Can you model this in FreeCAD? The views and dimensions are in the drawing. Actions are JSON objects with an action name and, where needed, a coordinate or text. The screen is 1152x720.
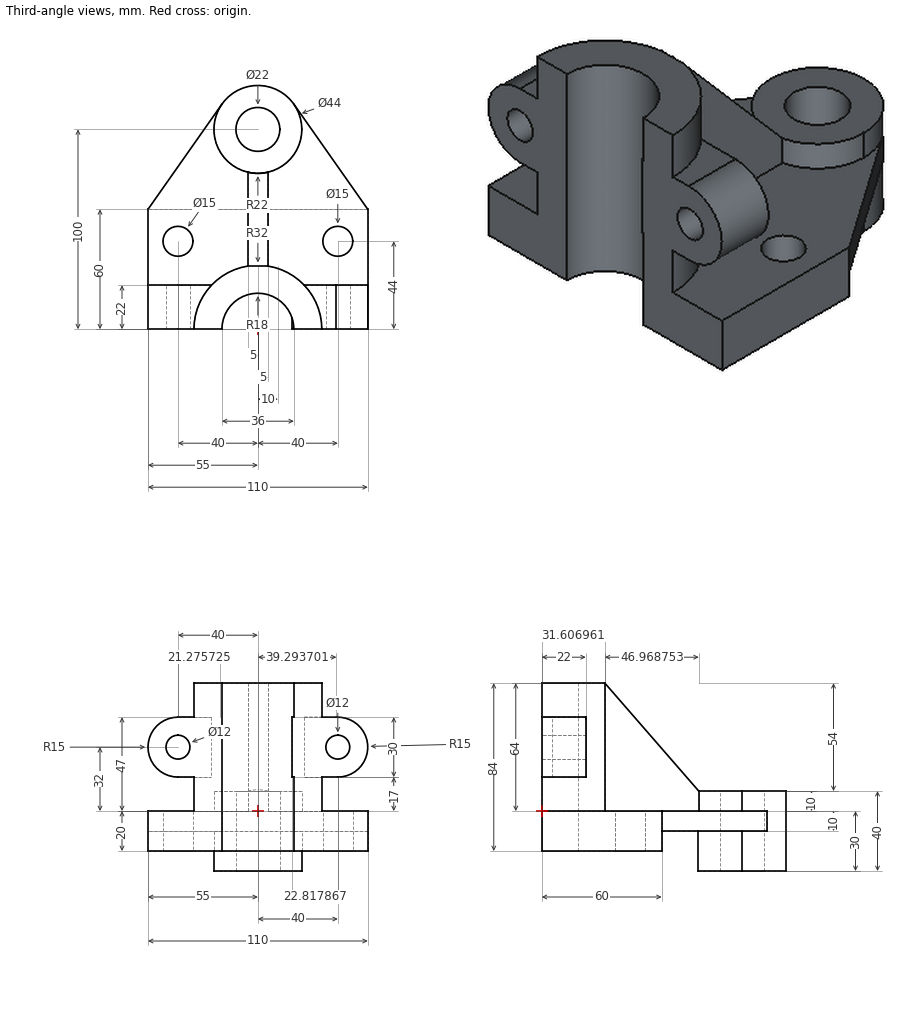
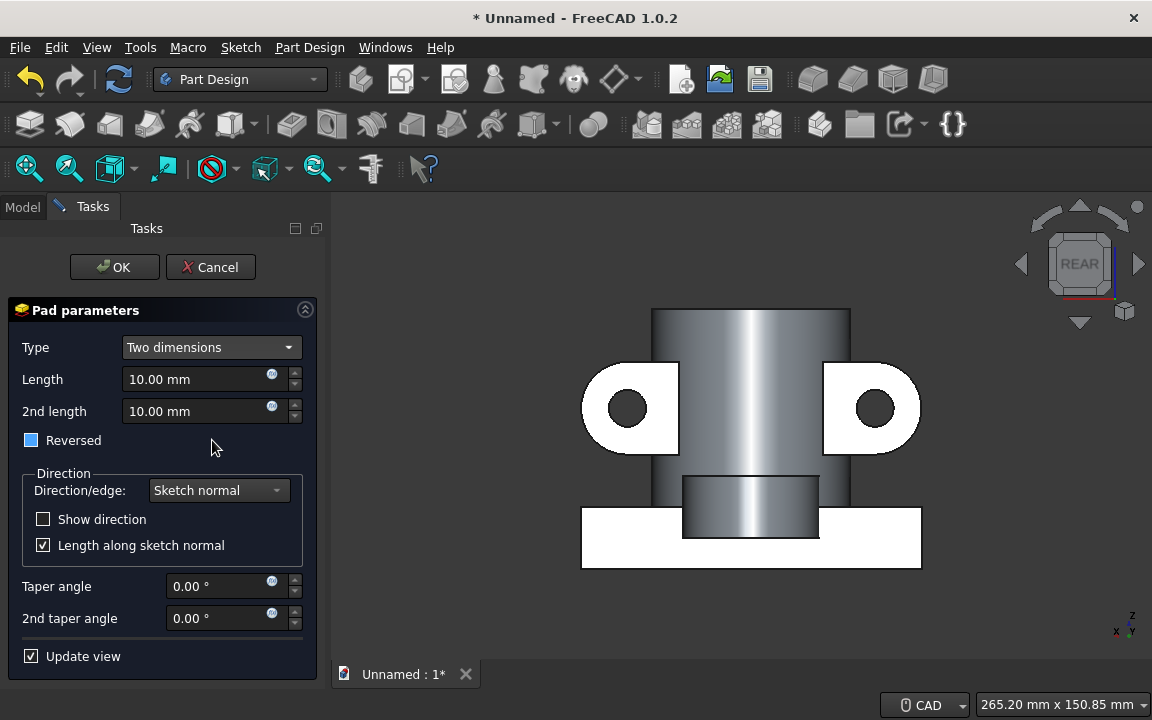
{"action": "triple_click", "coordinate": [204, 379]}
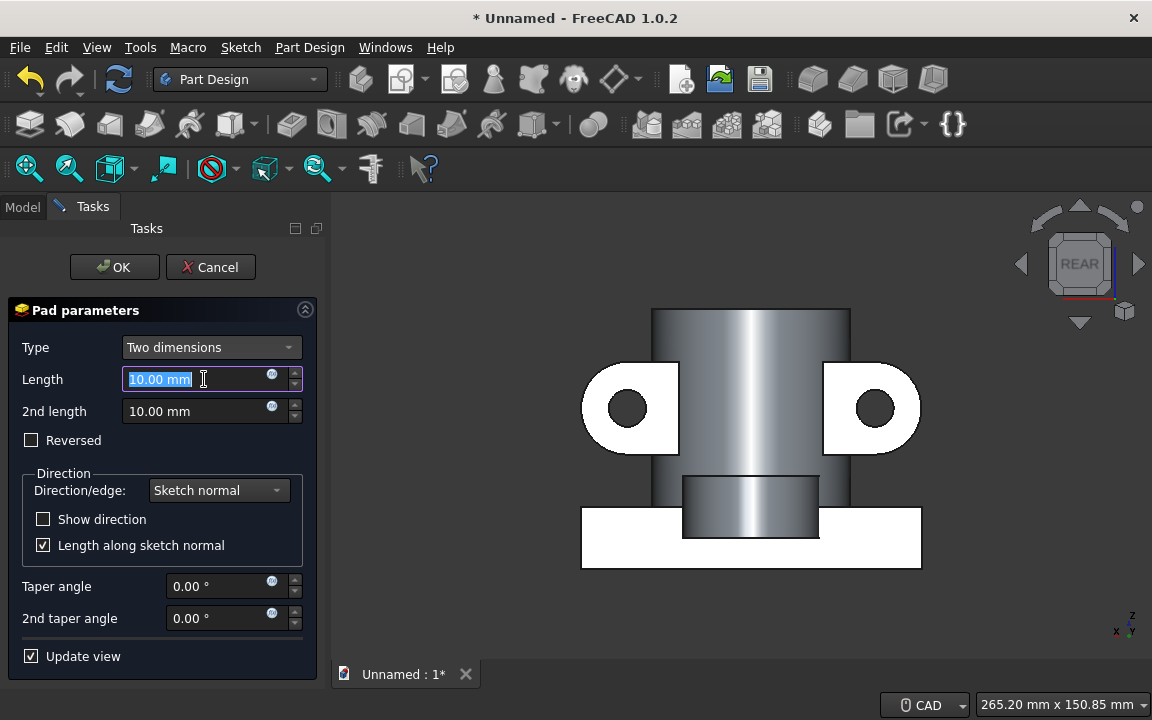
{"action": "type", "text": "10"}
{"action": "key", "text": "Tab"}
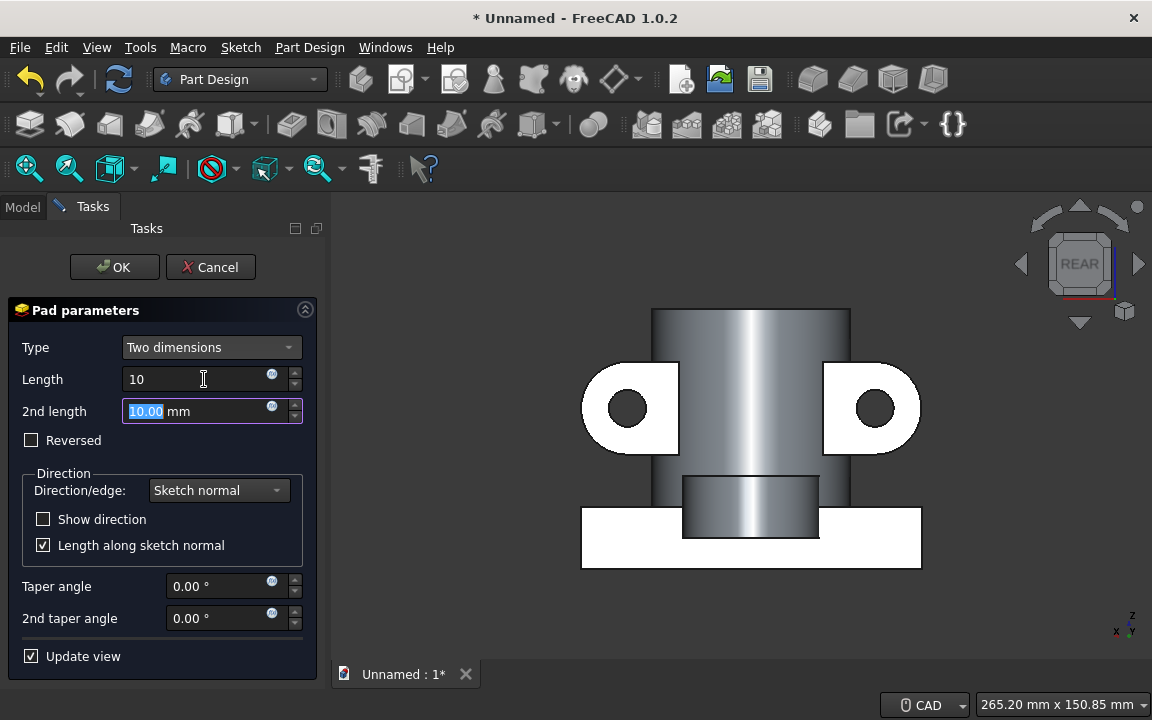
{"action": "type", "text": "30"}
{"action": "key", "text": "Tab"}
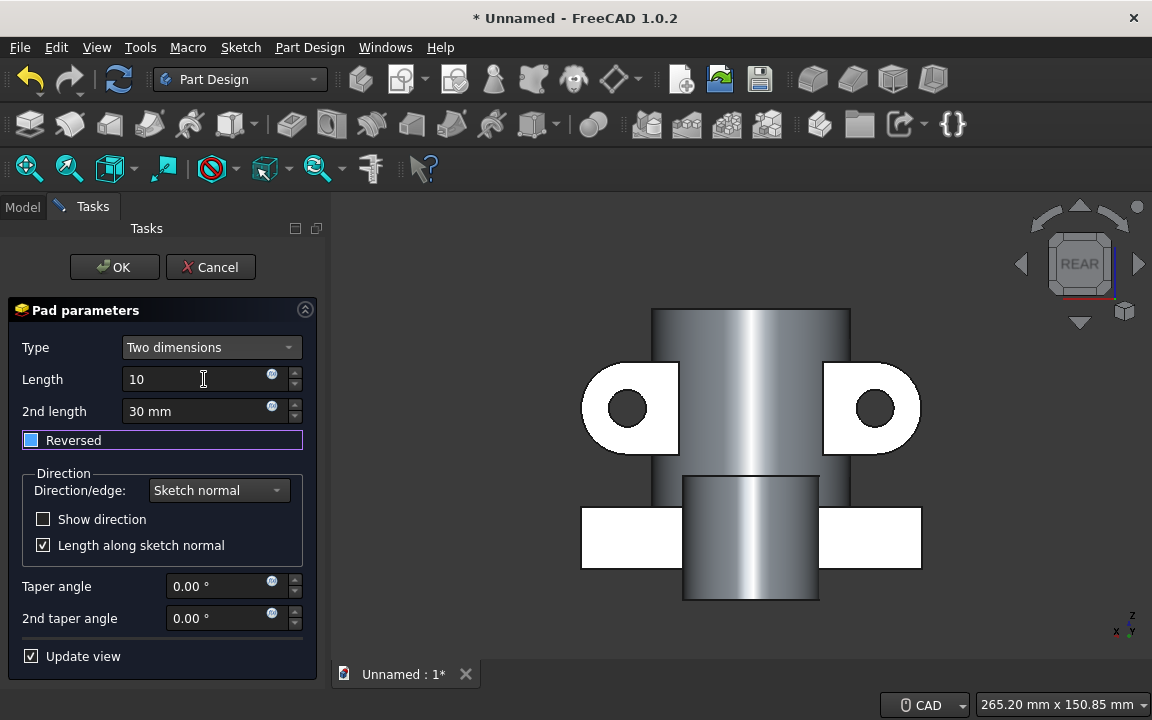
{"action": "left_click", "coordinate": [115, 267]}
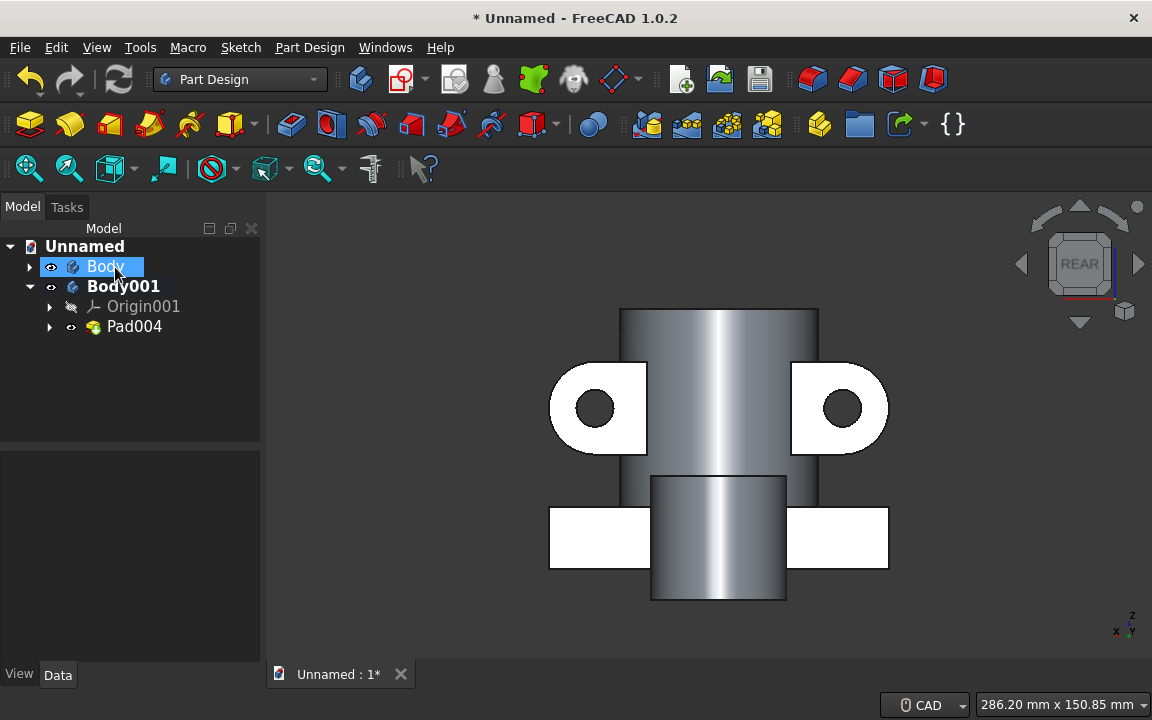
{"action": "left_click", "coordinate": [30, 170]}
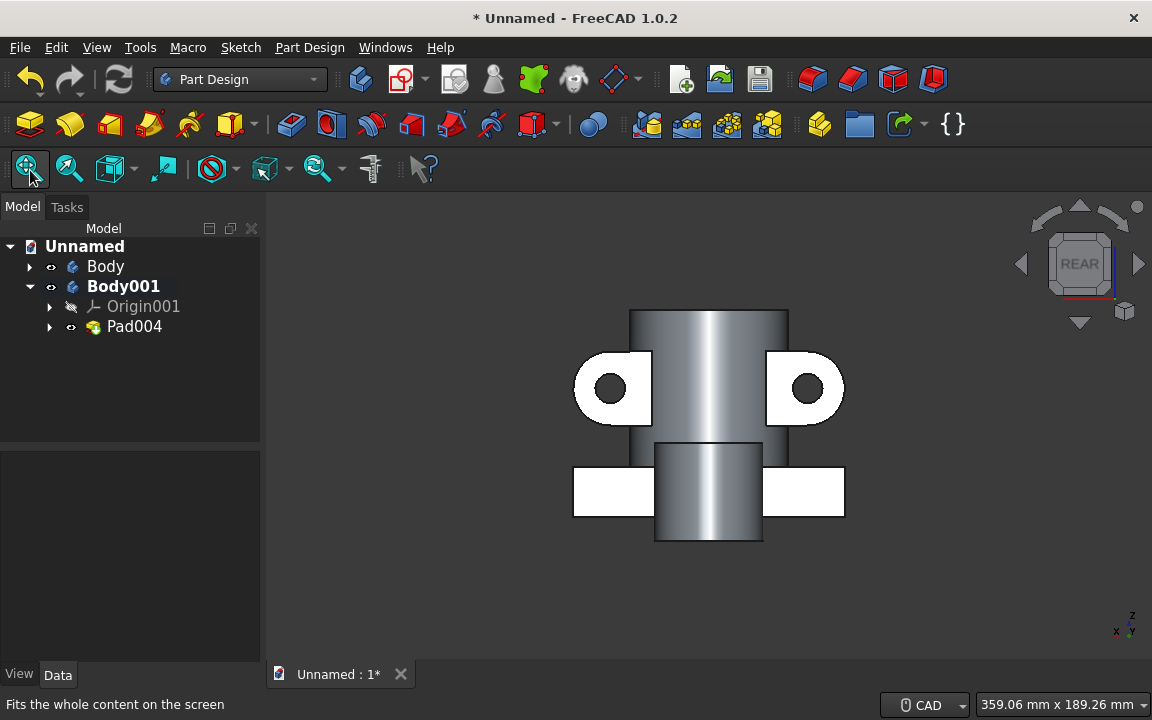
{"action": "double_click", "coordinate": [96, 267]}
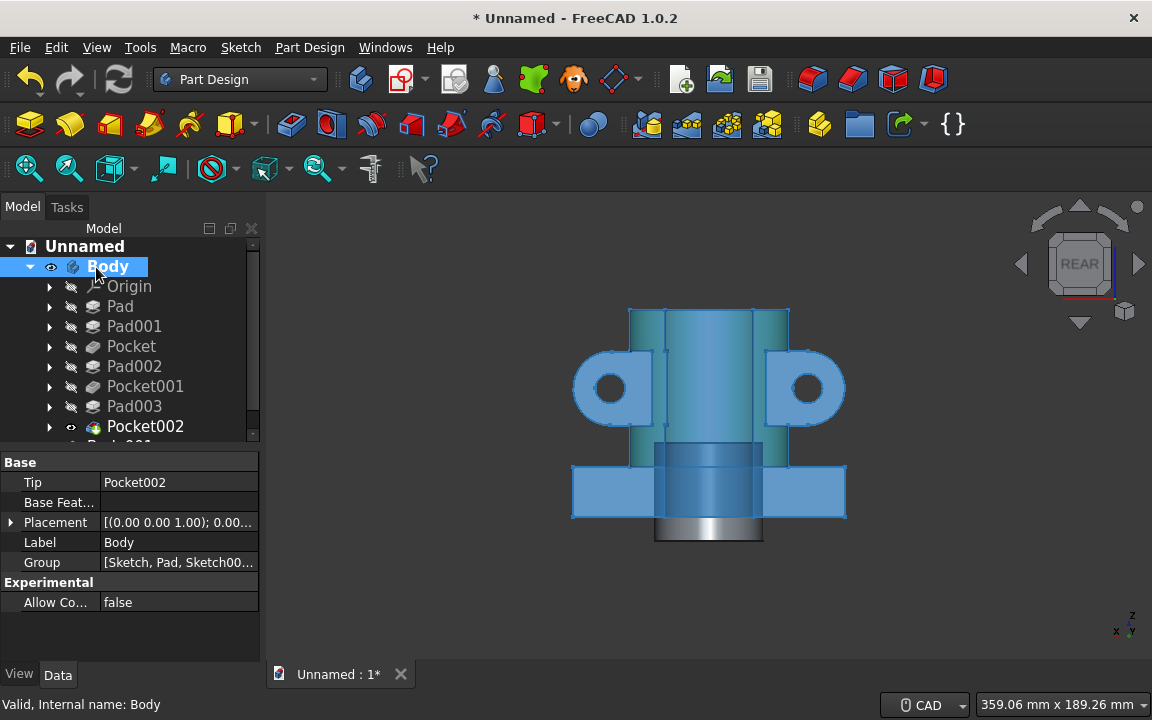
{"action": "left_click", "coordinate": [96, 267]}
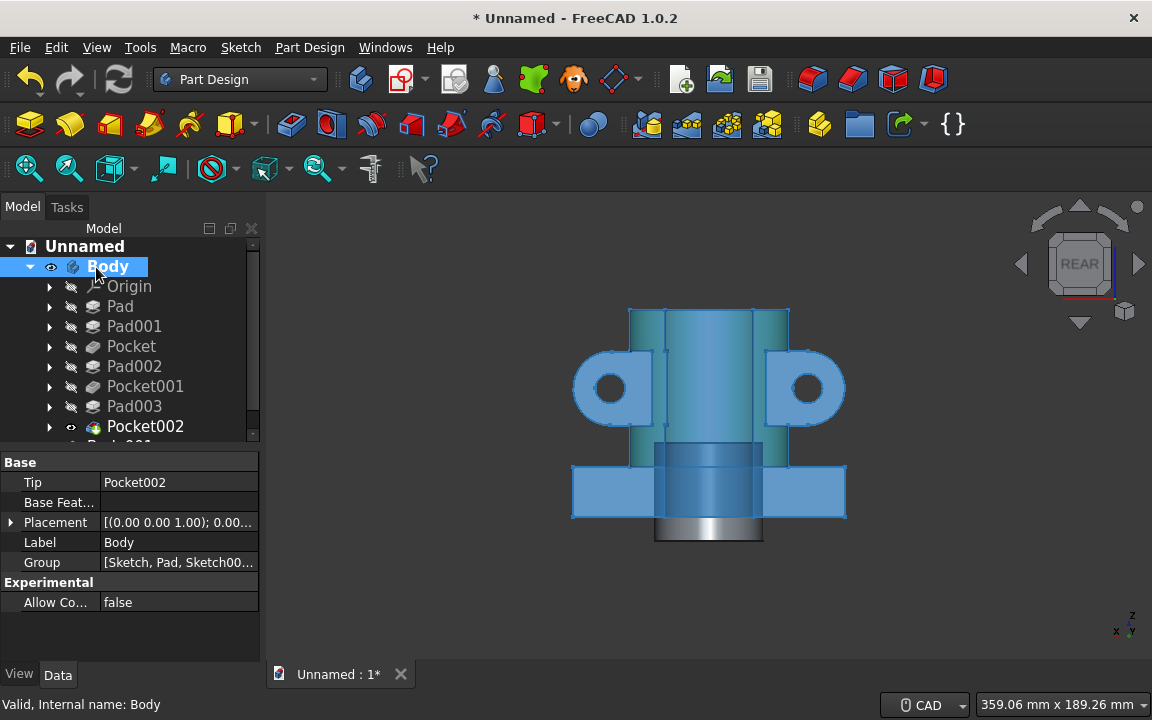
{"action": "left_click", "coordinate": [146, 602]}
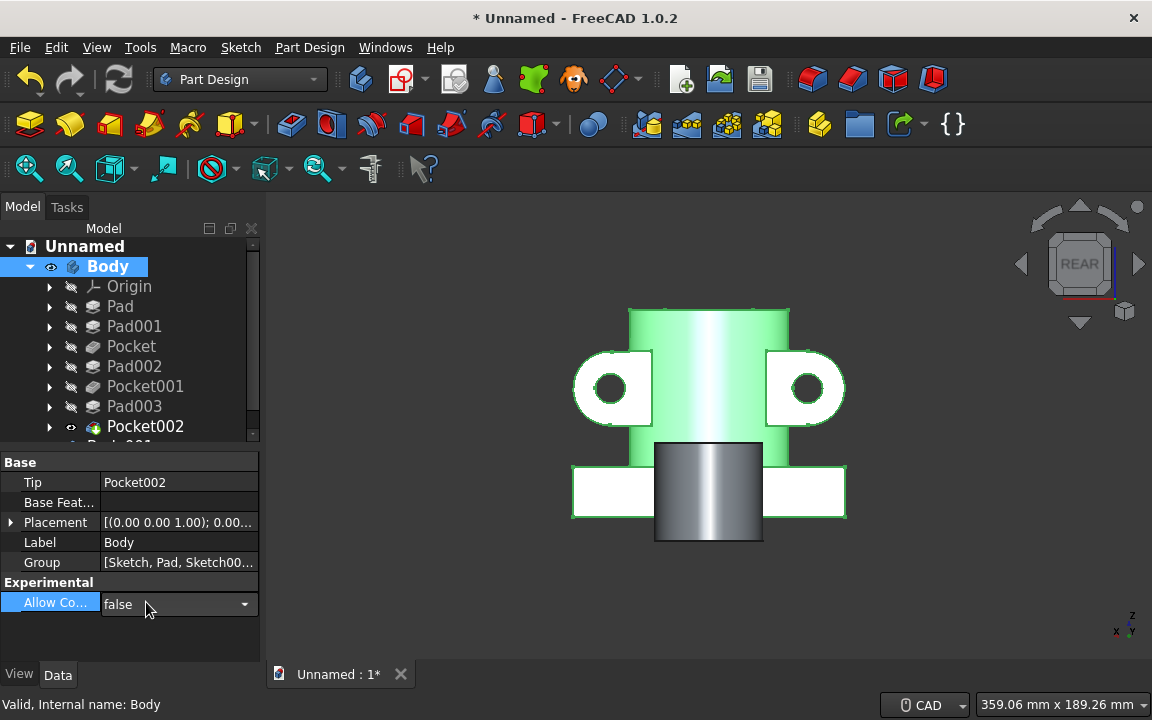
{"action": "left_click", "coordinate": [146, 602]}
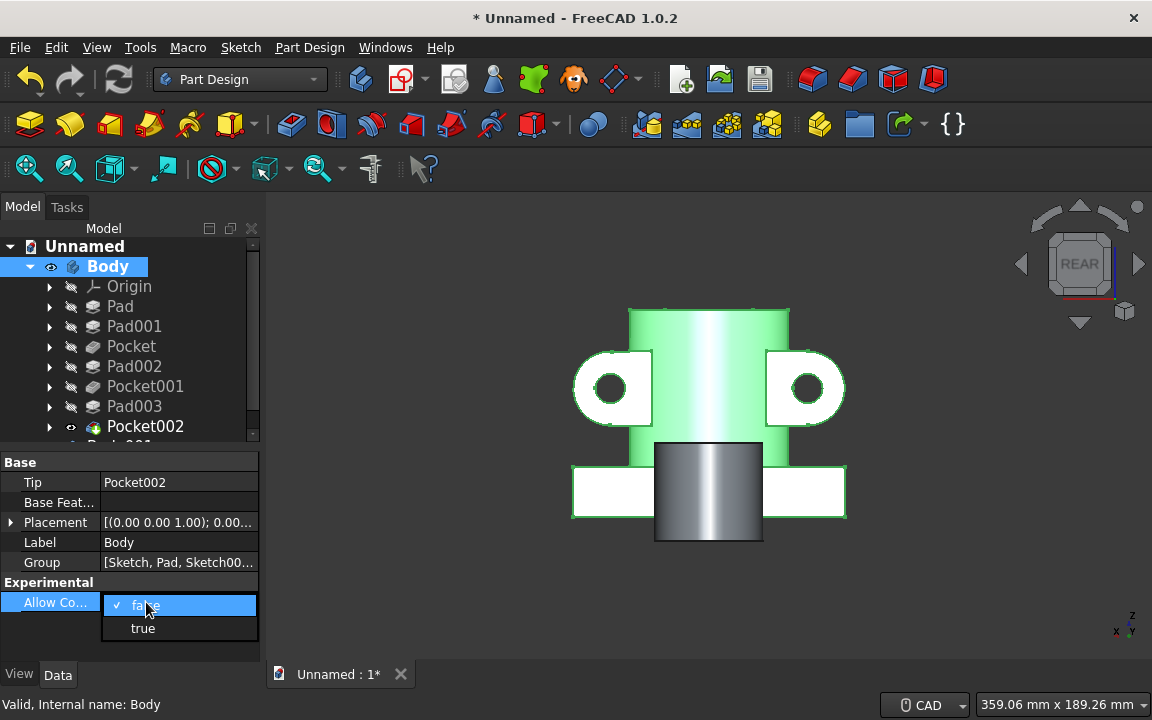
{"action": "left_click", "coordinate": [179, 628]}
{"action": "key", "text": "Return"}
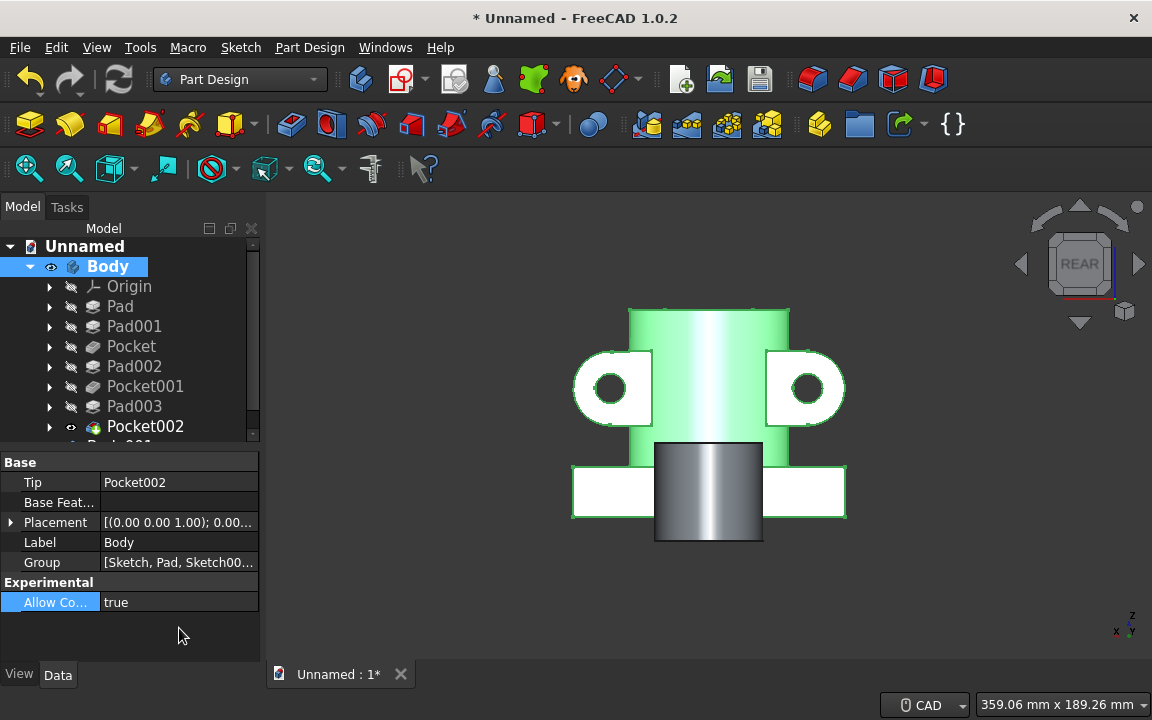
{"action": "scroll", "coordinate": [100, 342], "scroll_direction": "down", "scroll_amount": 3}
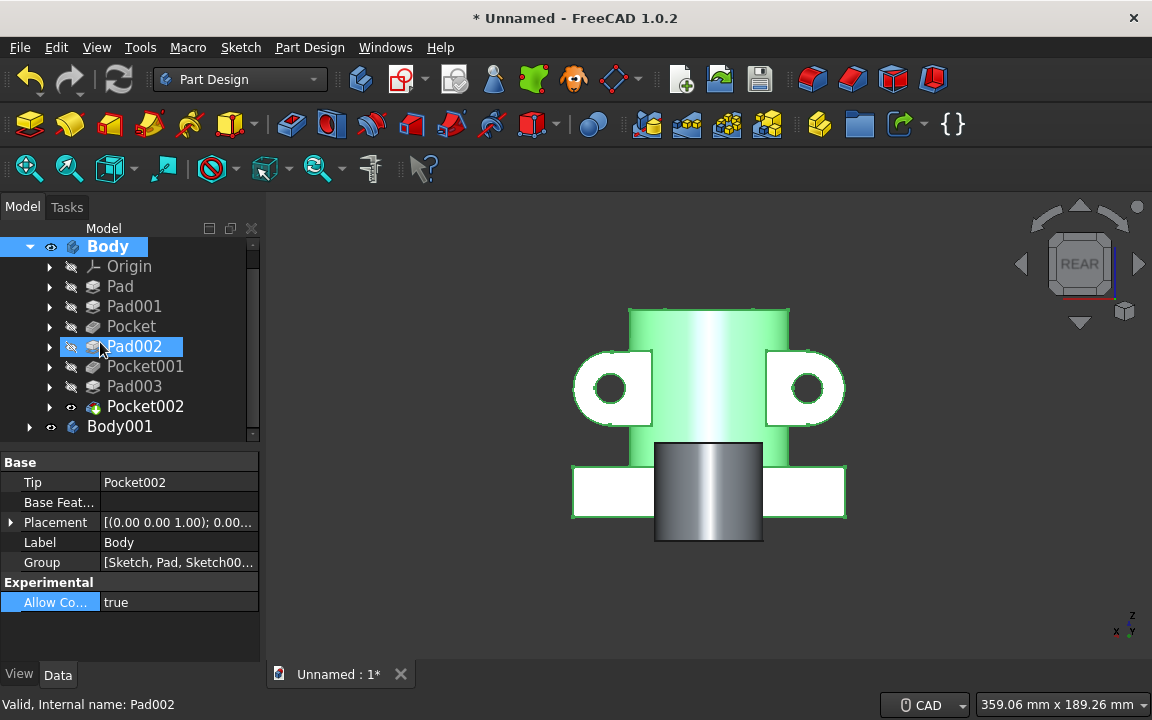
{"action": "left_click", "coordinate": [96, 427]}